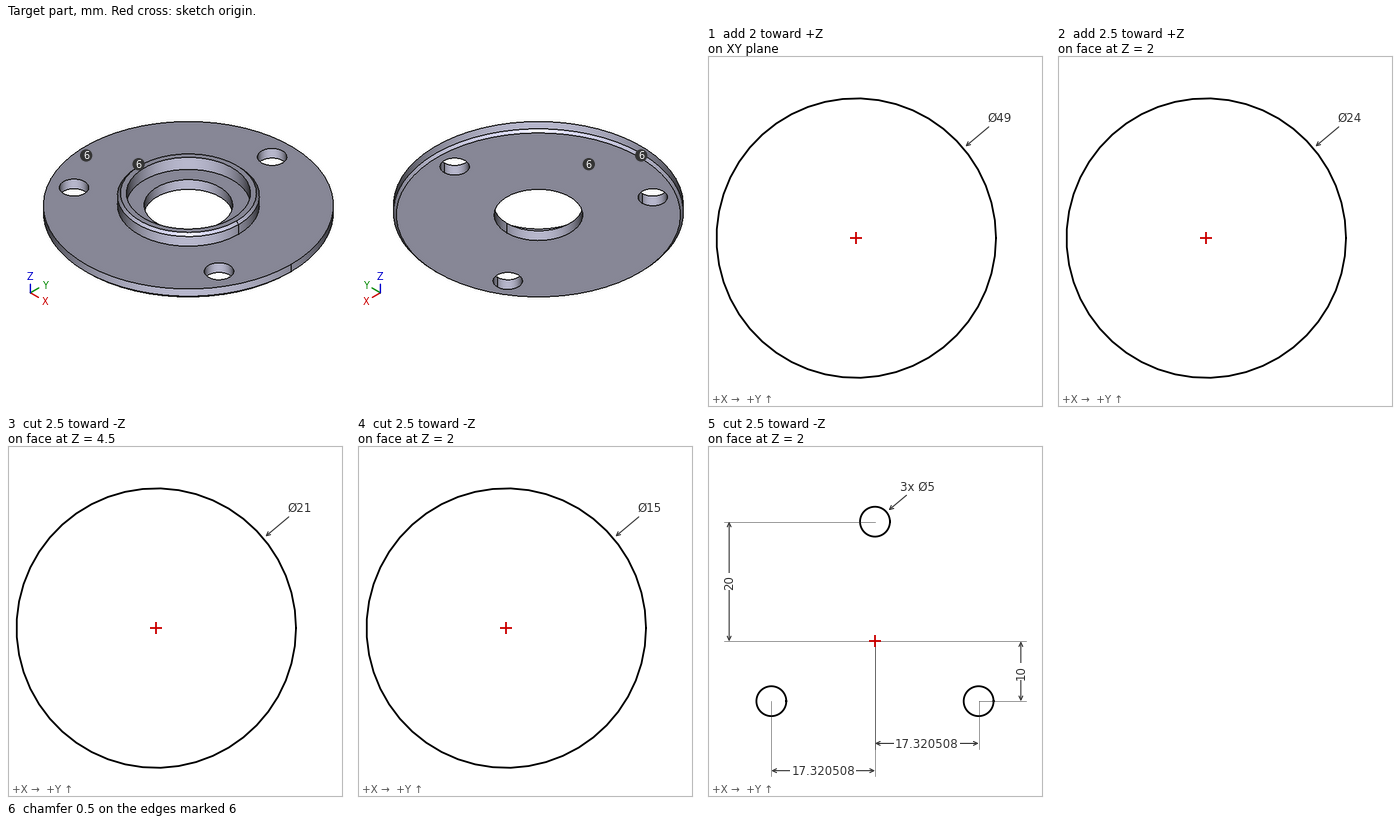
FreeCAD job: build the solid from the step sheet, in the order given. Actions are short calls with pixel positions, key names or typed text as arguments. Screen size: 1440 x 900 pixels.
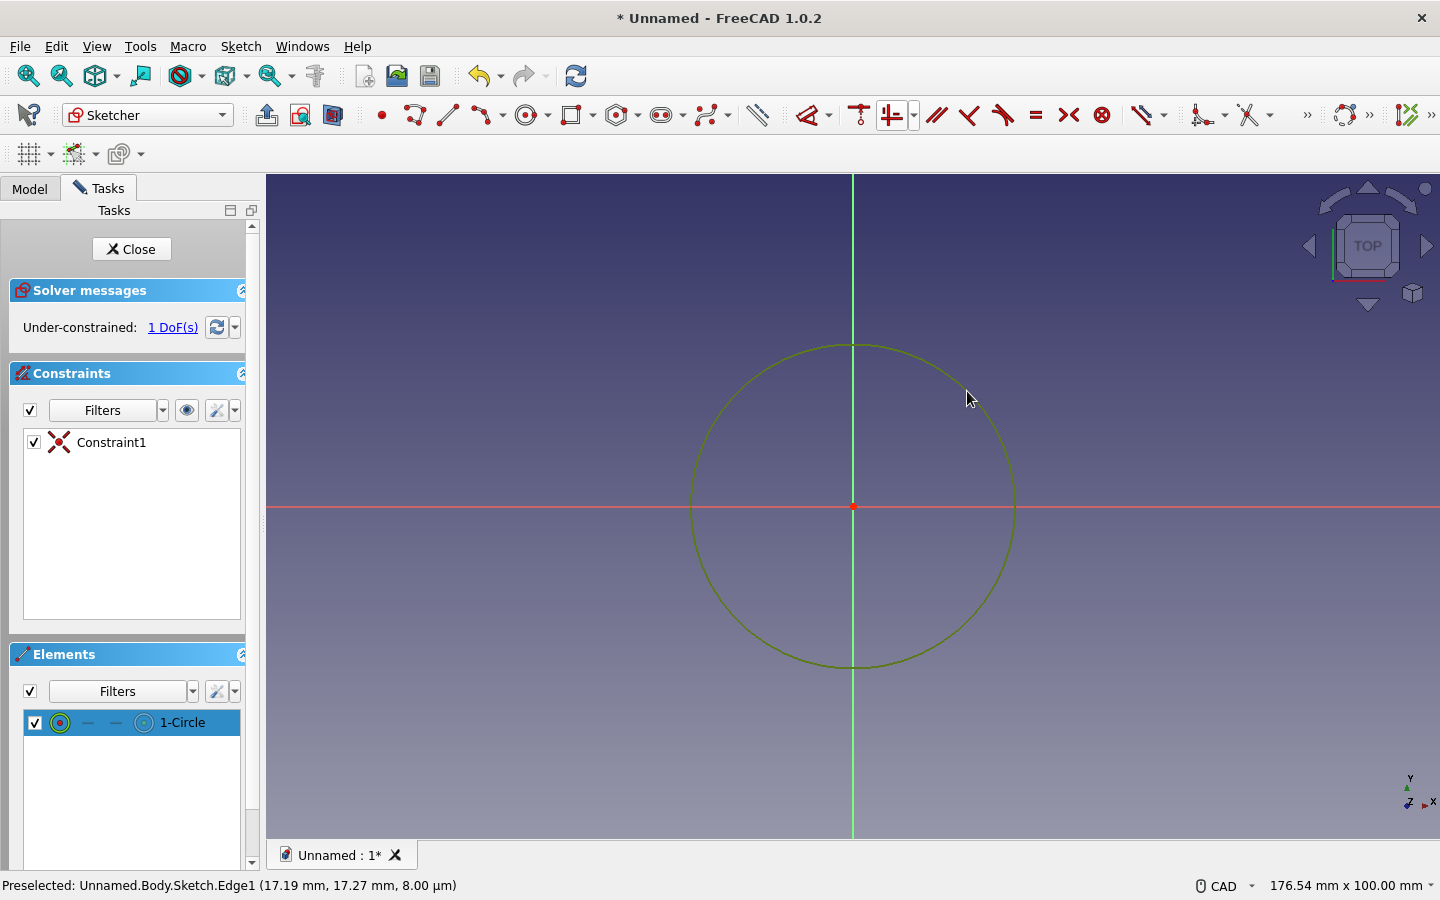
key(k)
key(o)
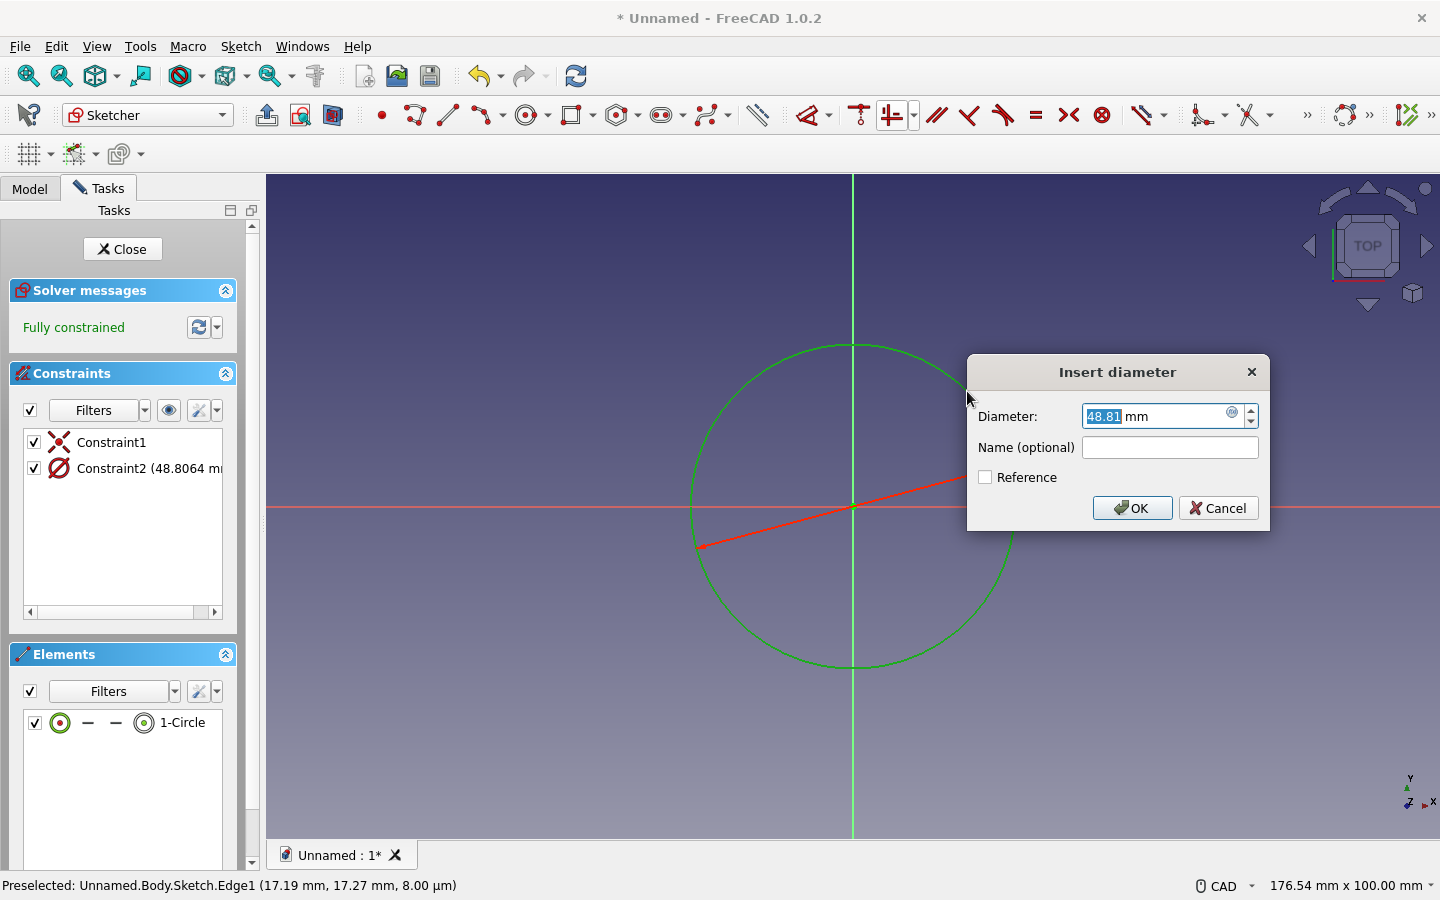
text(49)
key(Return)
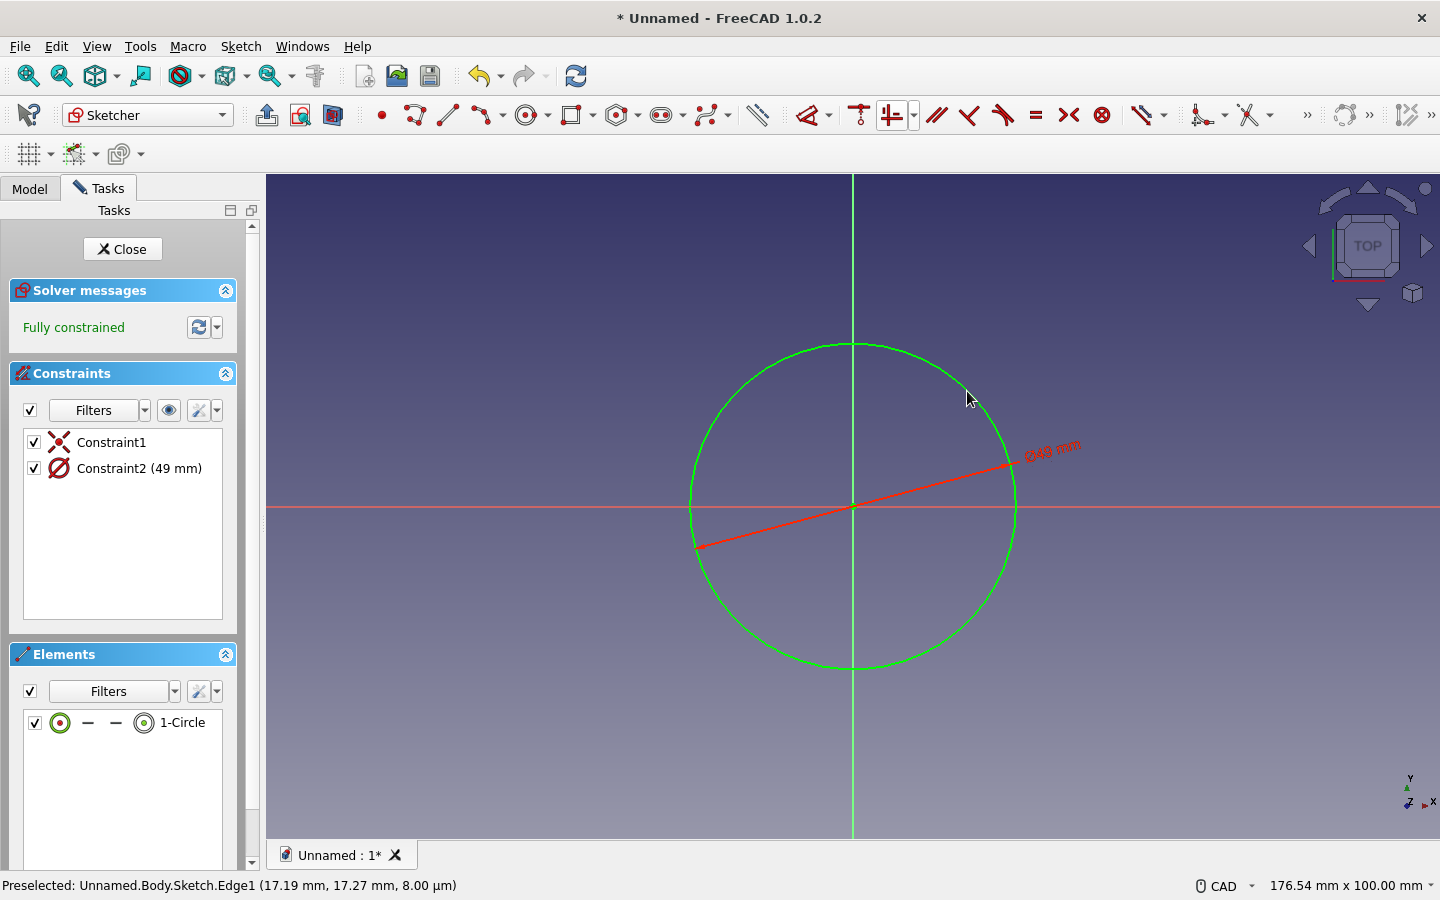
click(123, 249)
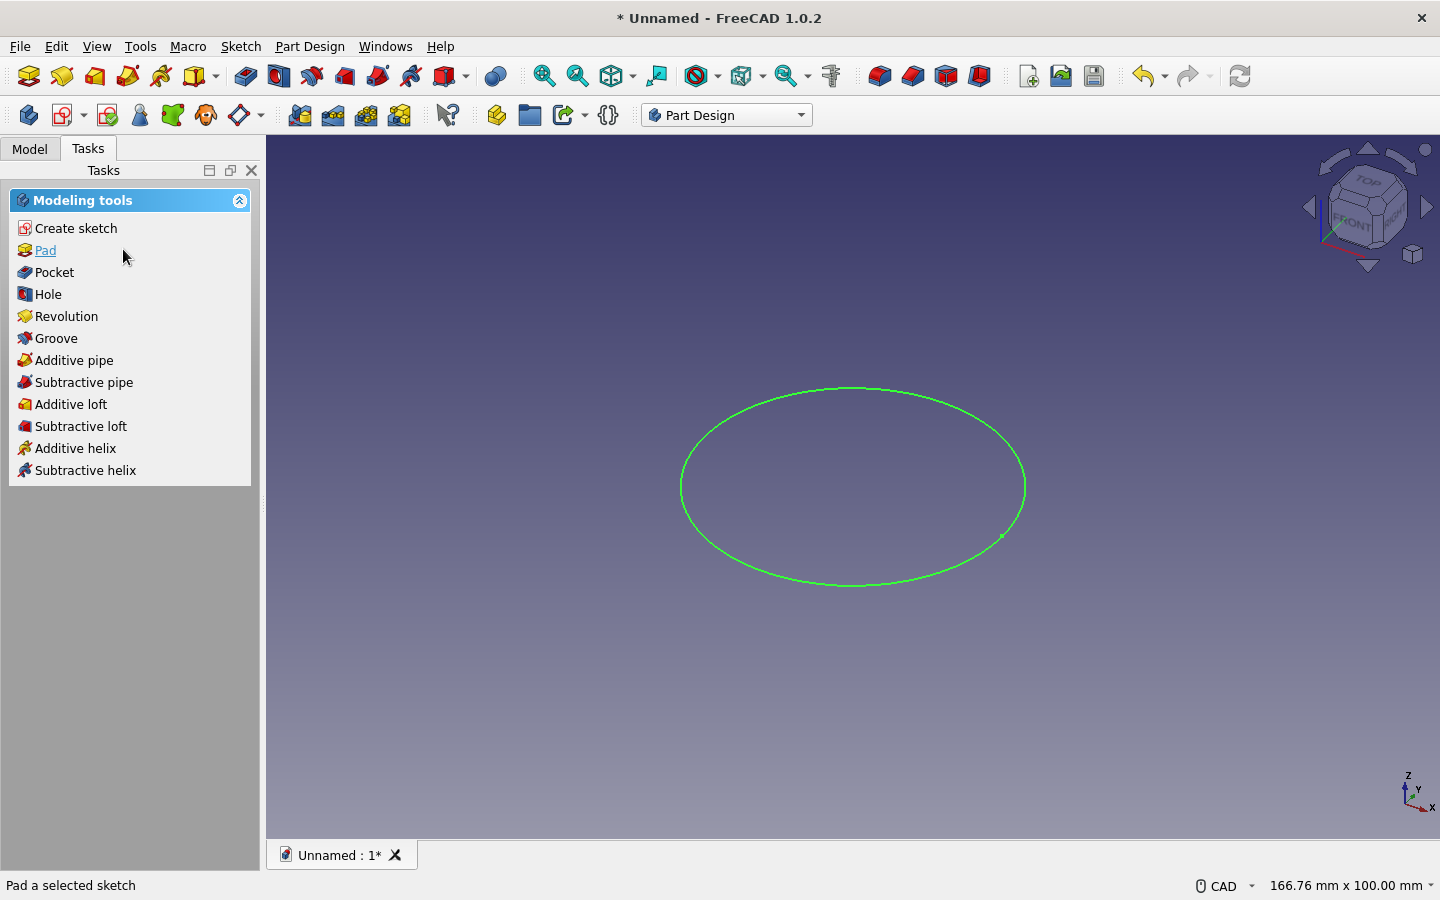
click(29, 76)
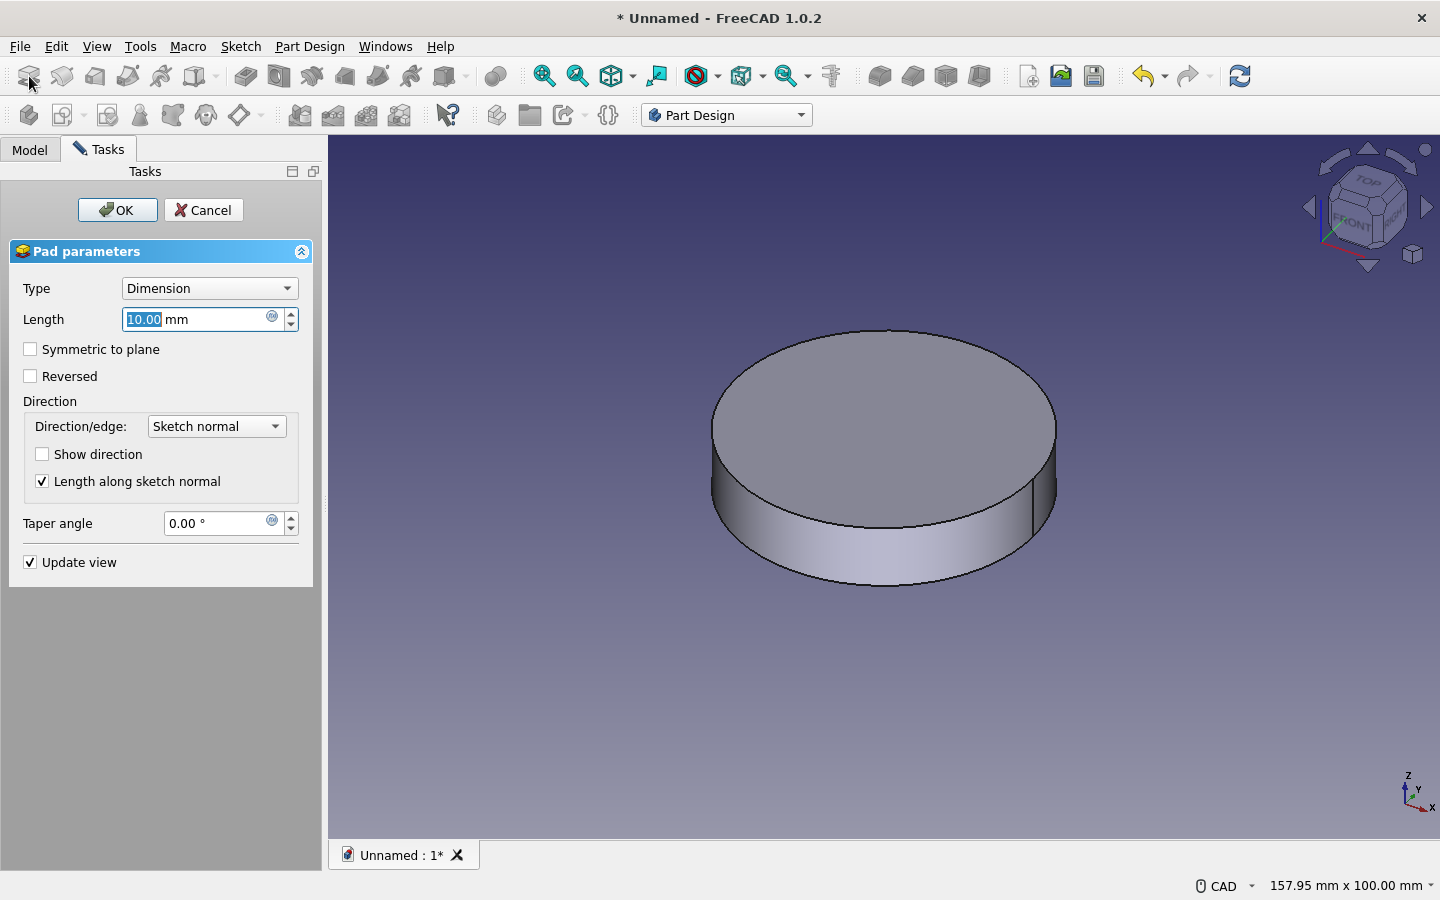
text(2)
key(Tab)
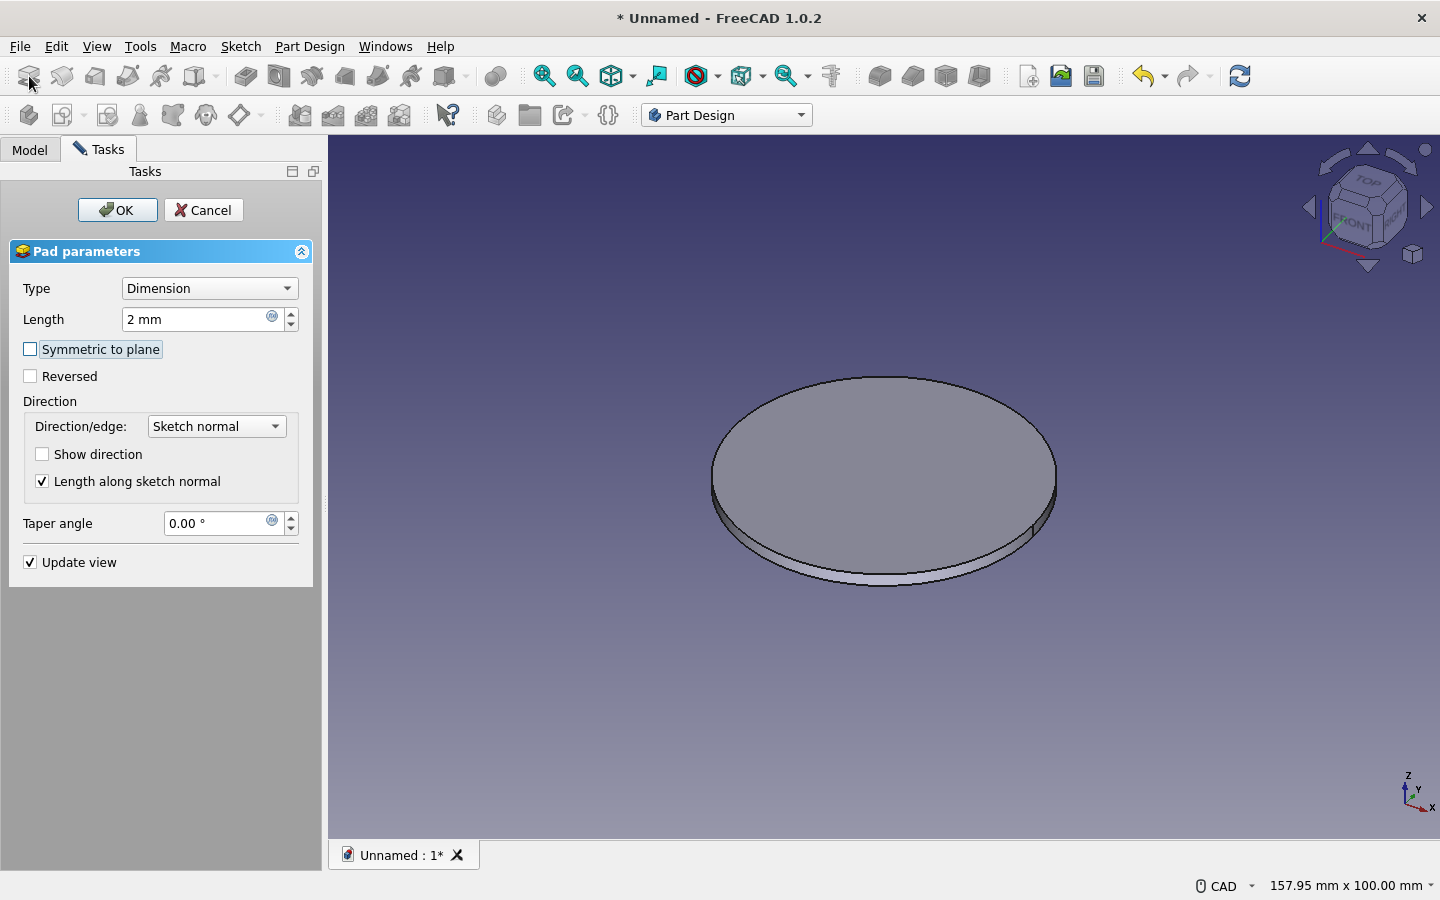
click(118, 210)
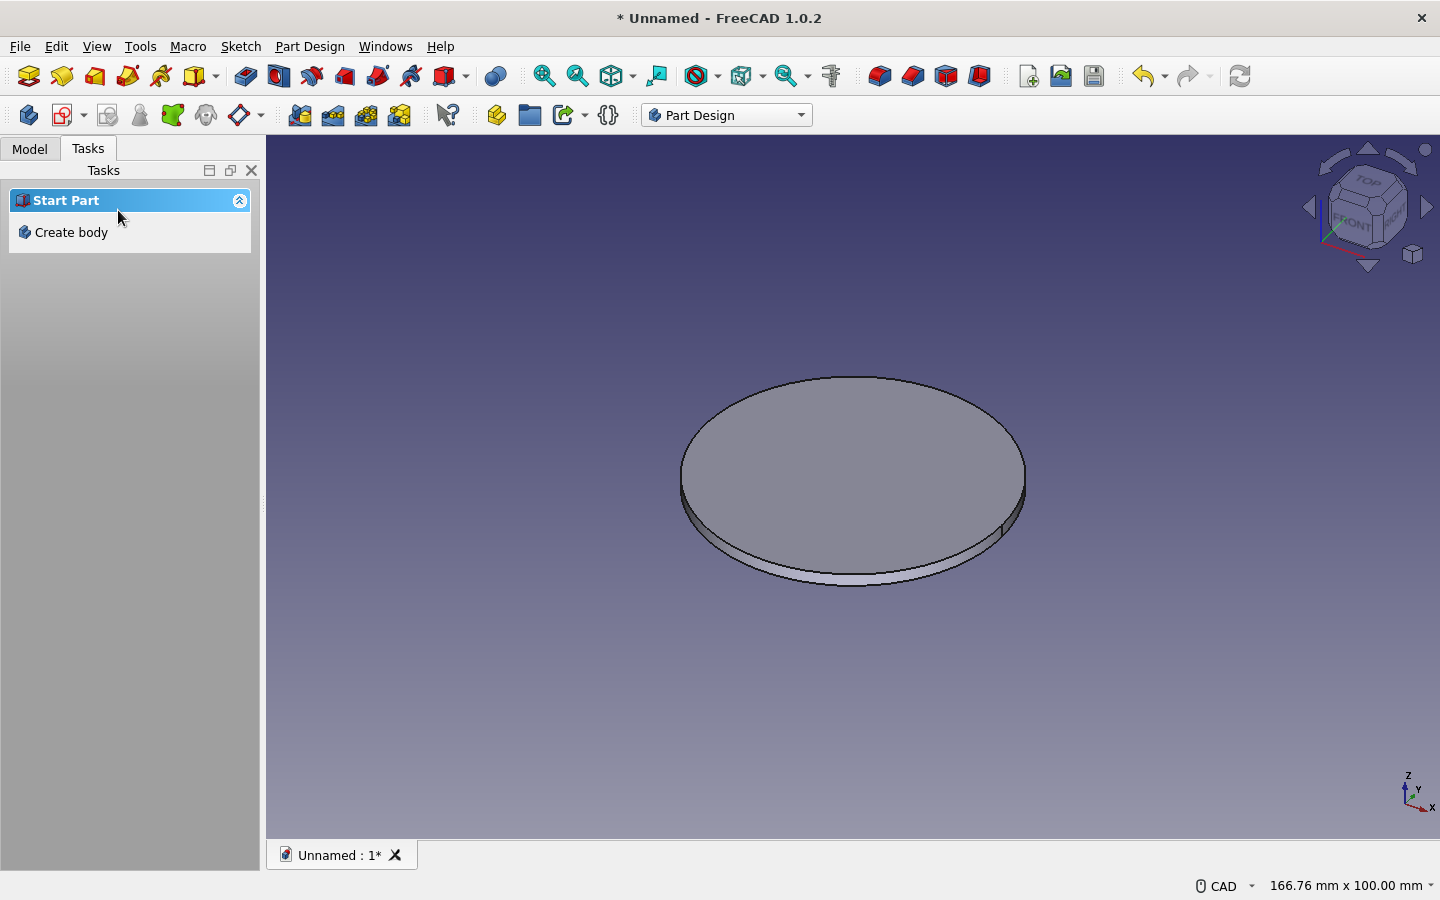
click(545, 76)